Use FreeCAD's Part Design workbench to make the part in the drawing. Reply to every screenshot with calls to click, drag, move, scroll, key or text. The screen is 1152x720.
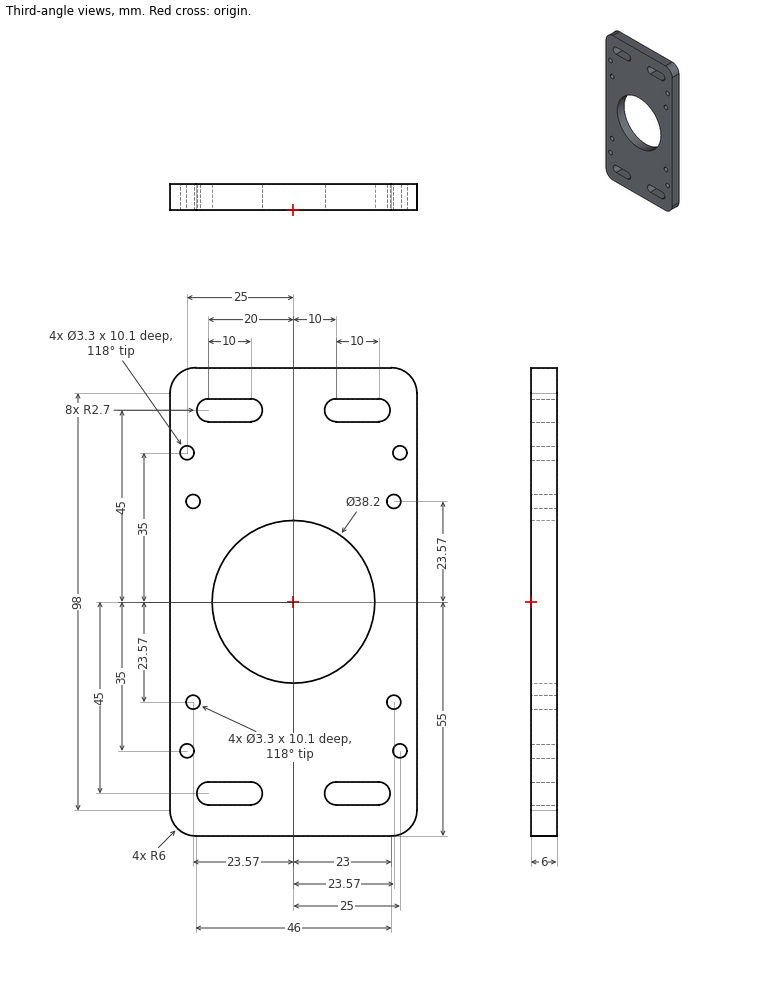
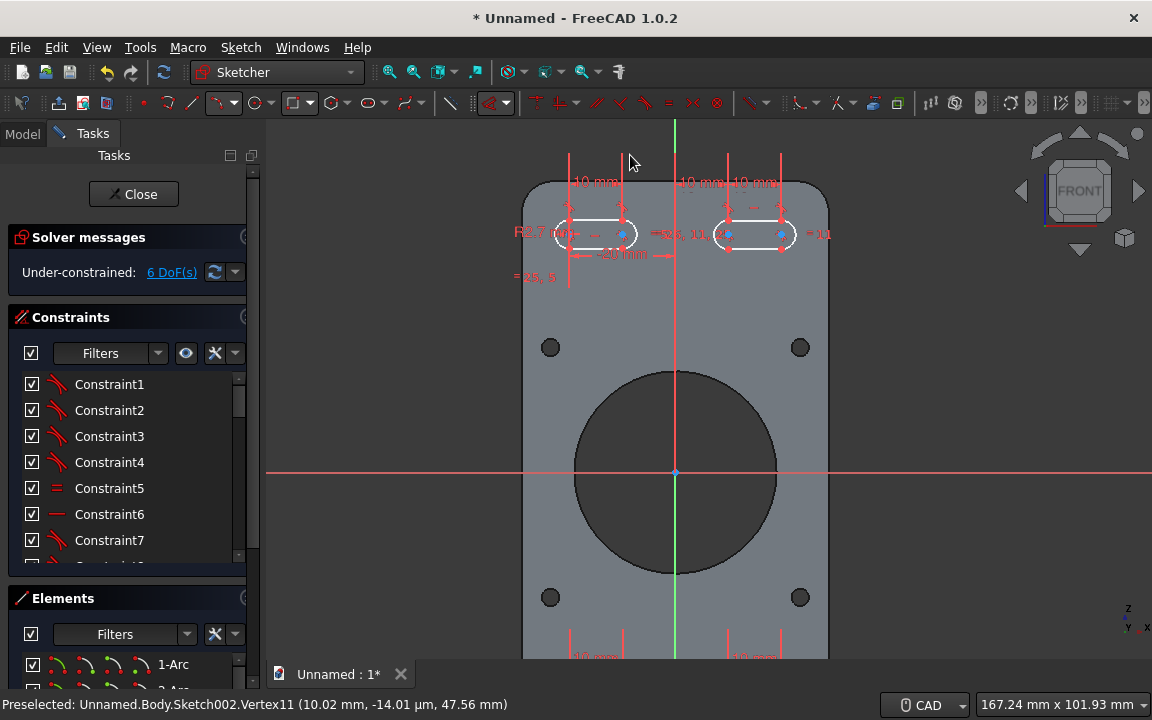
scroll(570, 219, down, 2)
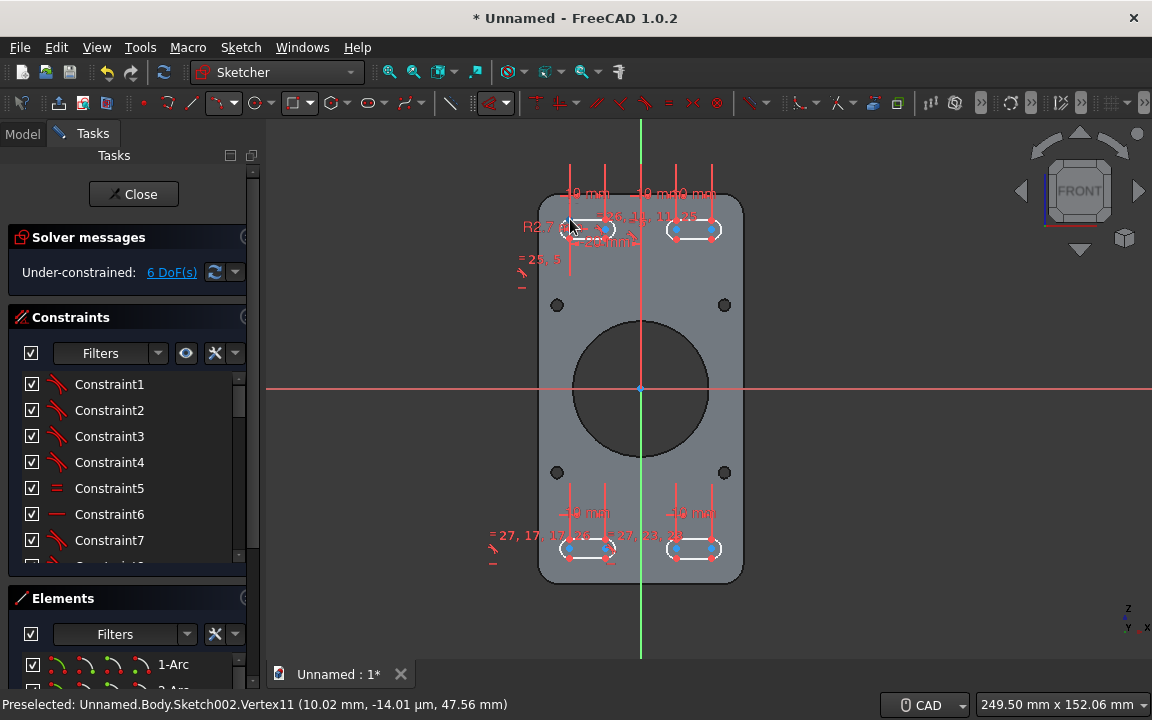
scroll(570, 539, up, 2)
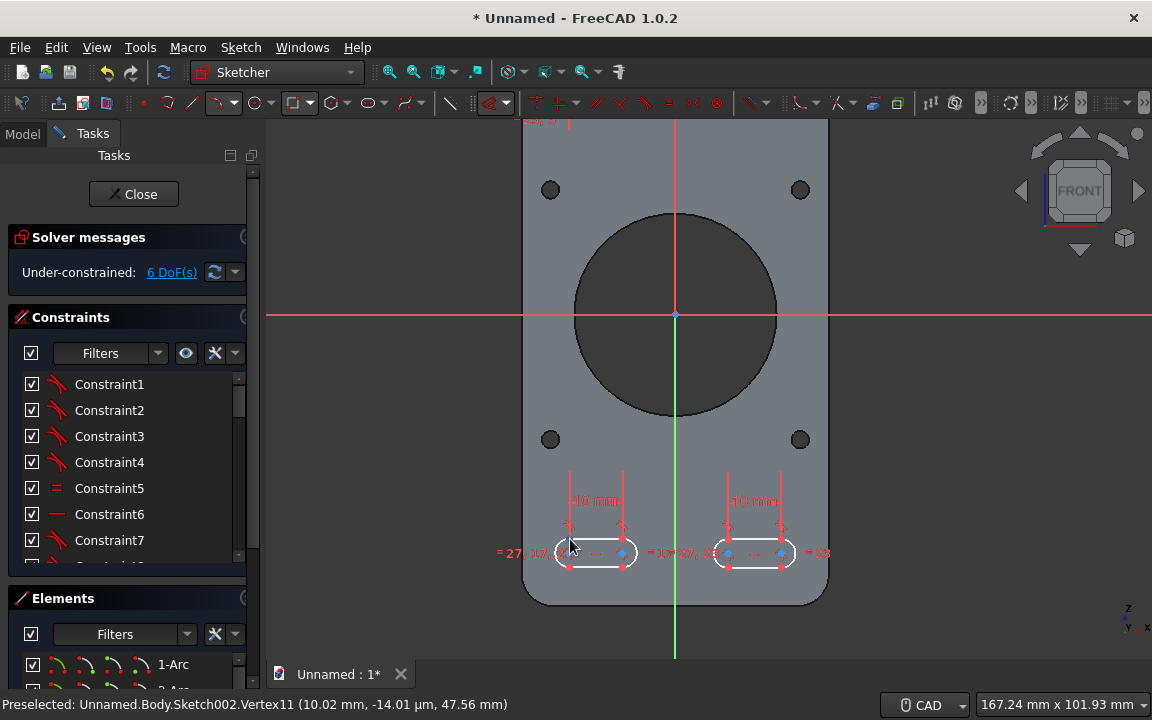
click(570, 539)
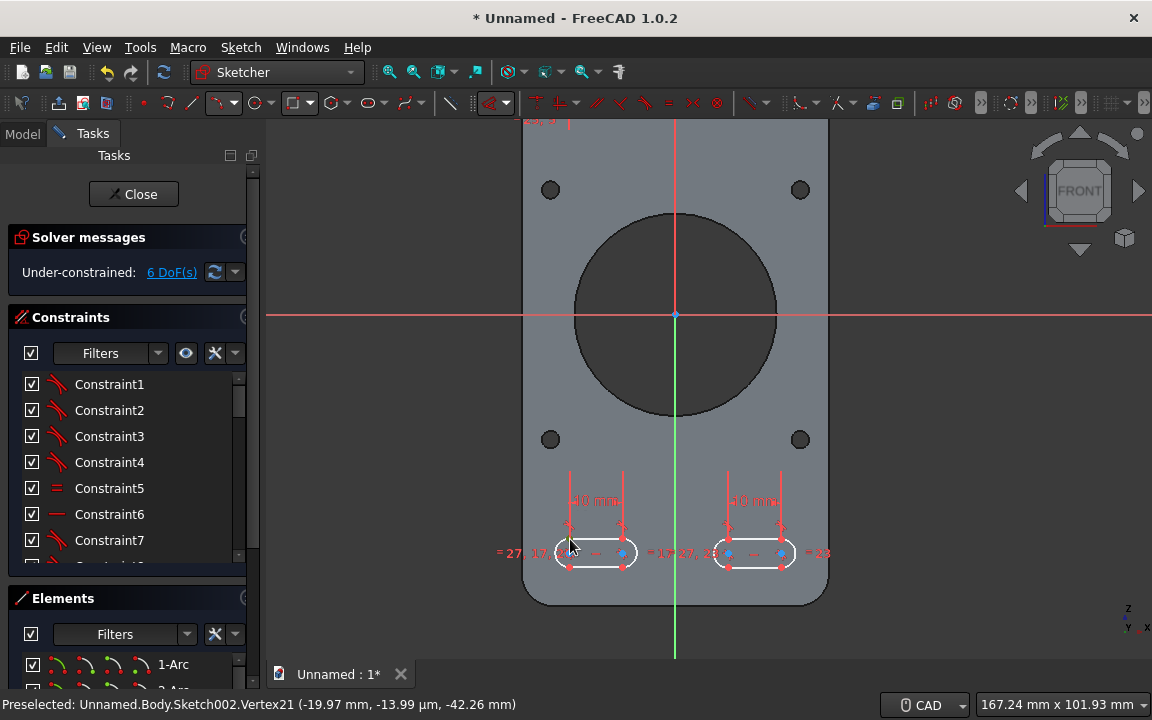
click(508, 104)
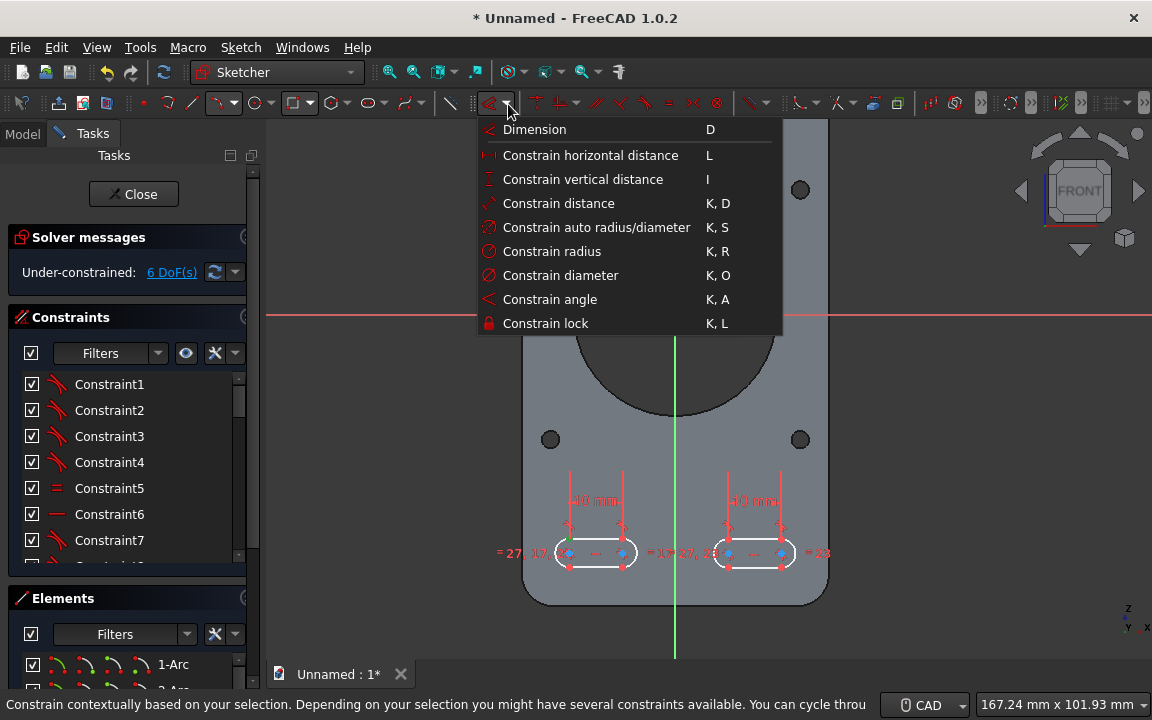
click(630, 155)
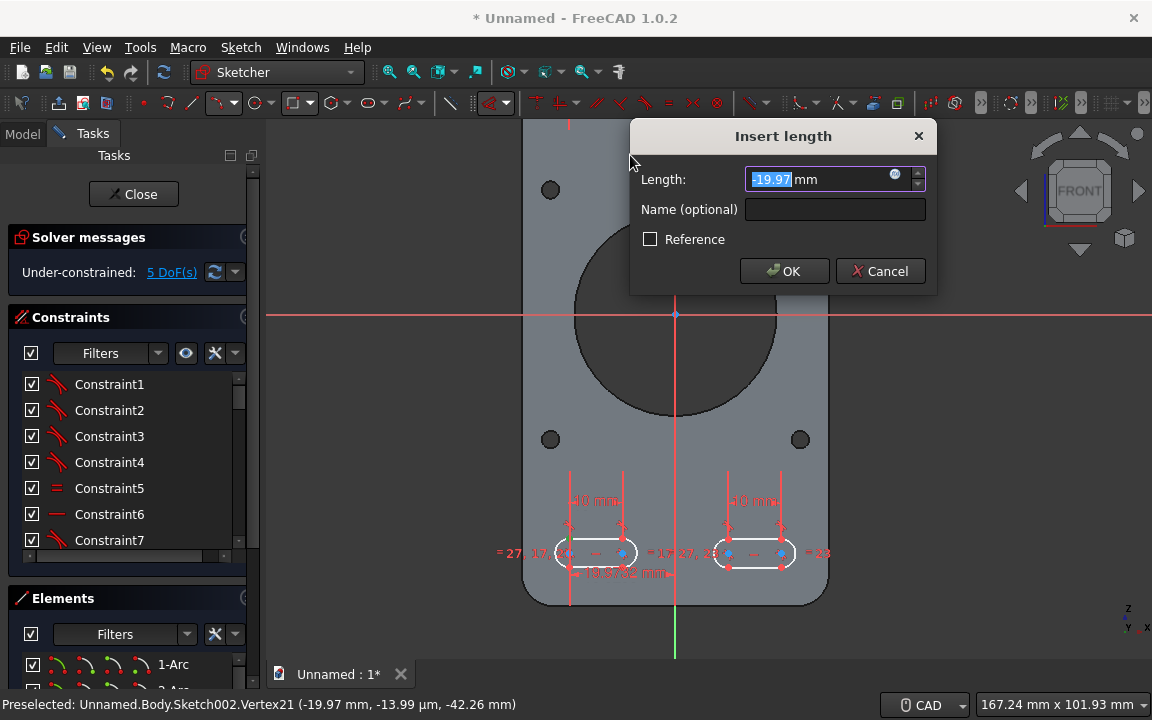
text(-20)
key(Return)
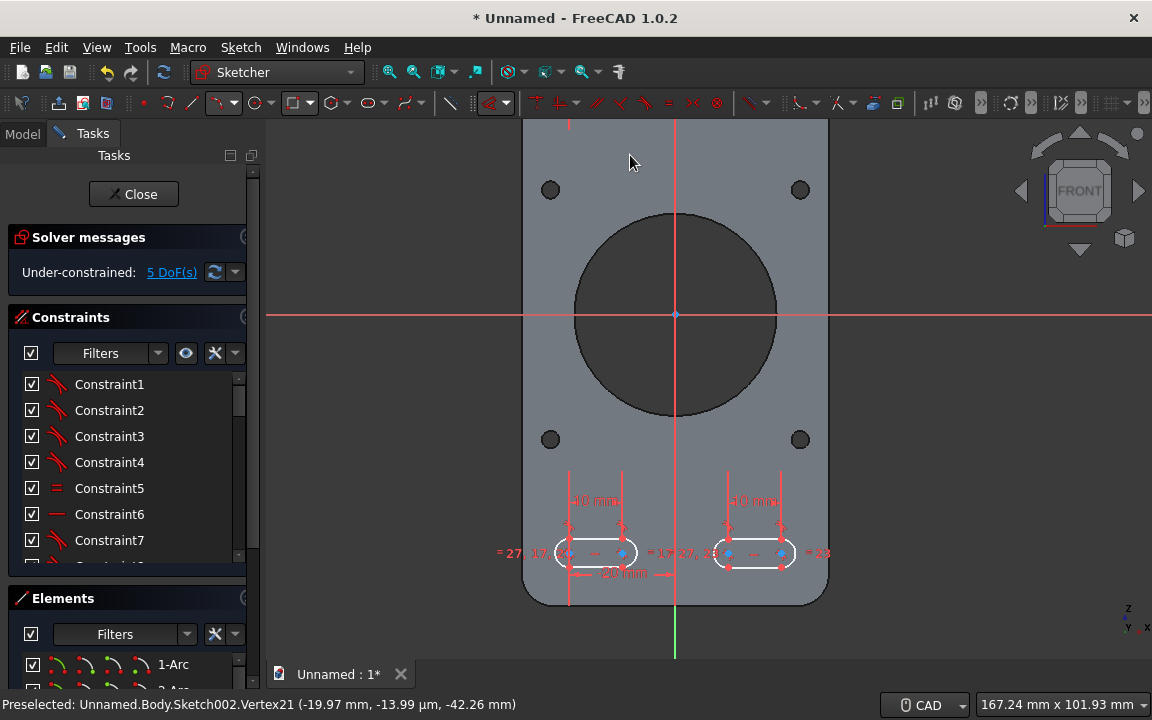
click(728, 539)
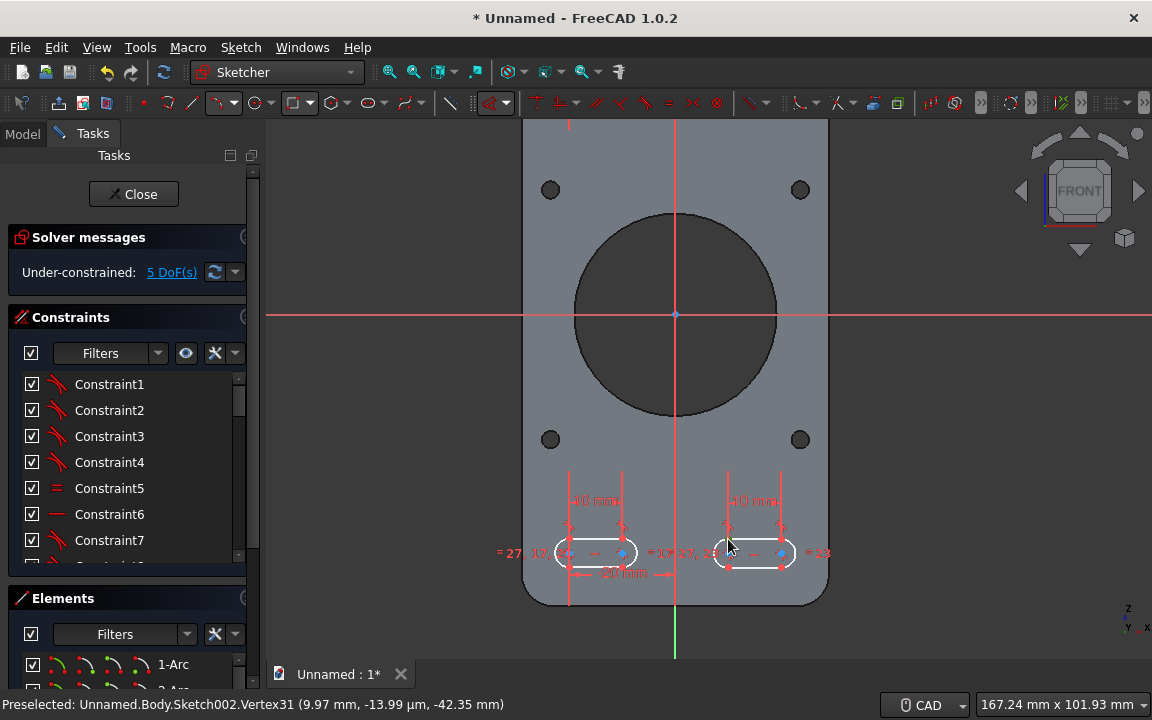
click(508, 104)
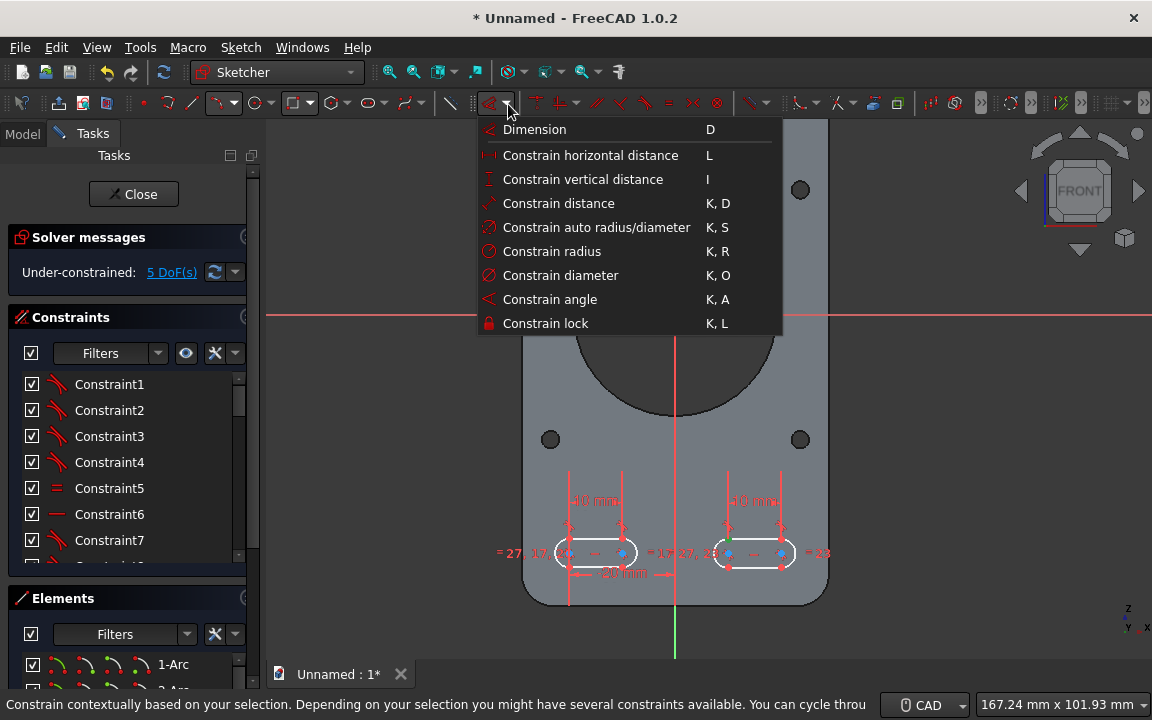
click(630, 155)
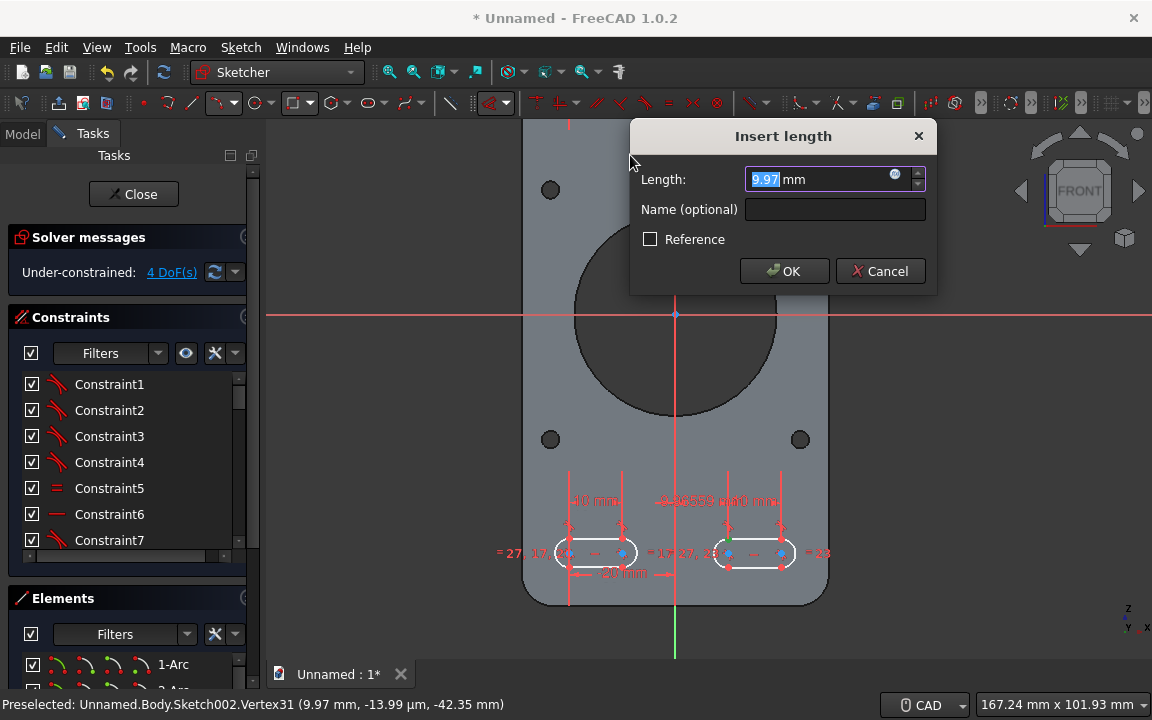
text(10)
key(Return)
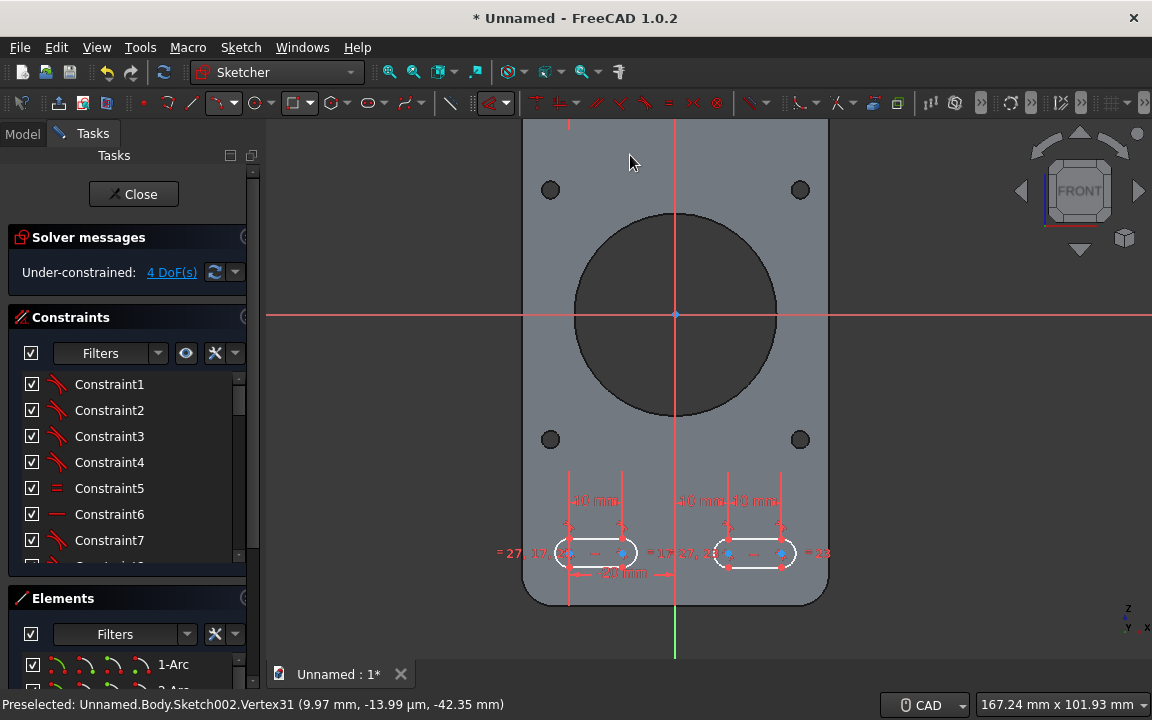
scroll(570, 540, down, 2)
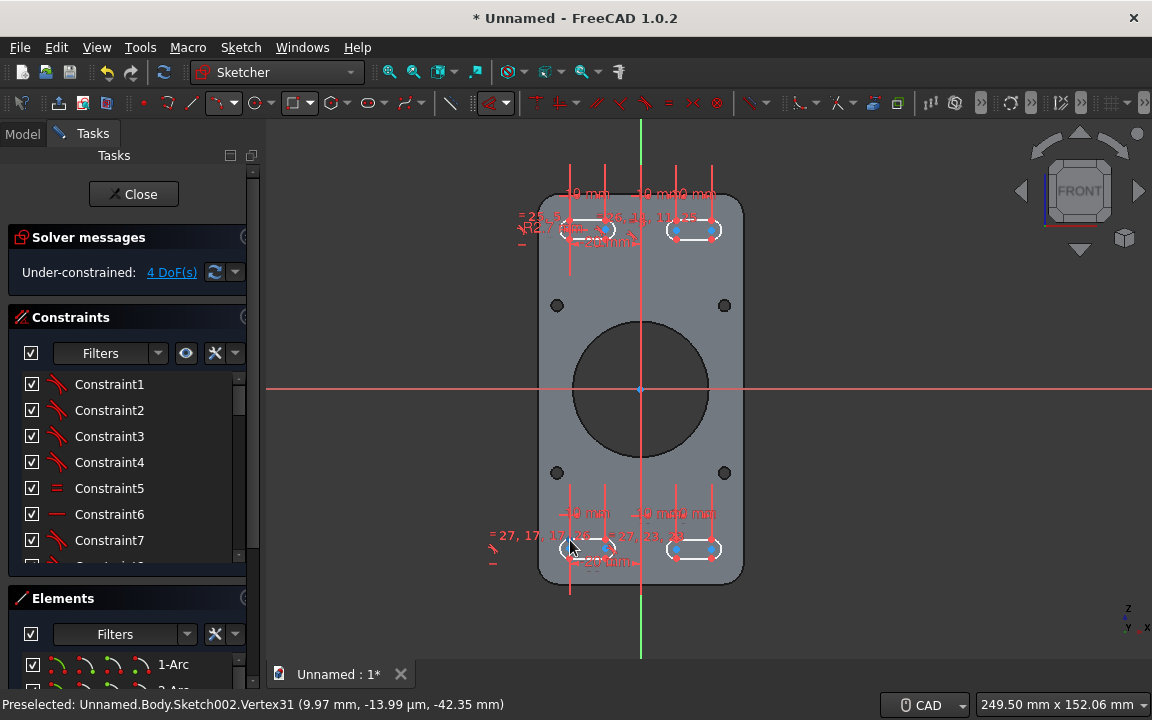
scroll(570, 230, up, 2)